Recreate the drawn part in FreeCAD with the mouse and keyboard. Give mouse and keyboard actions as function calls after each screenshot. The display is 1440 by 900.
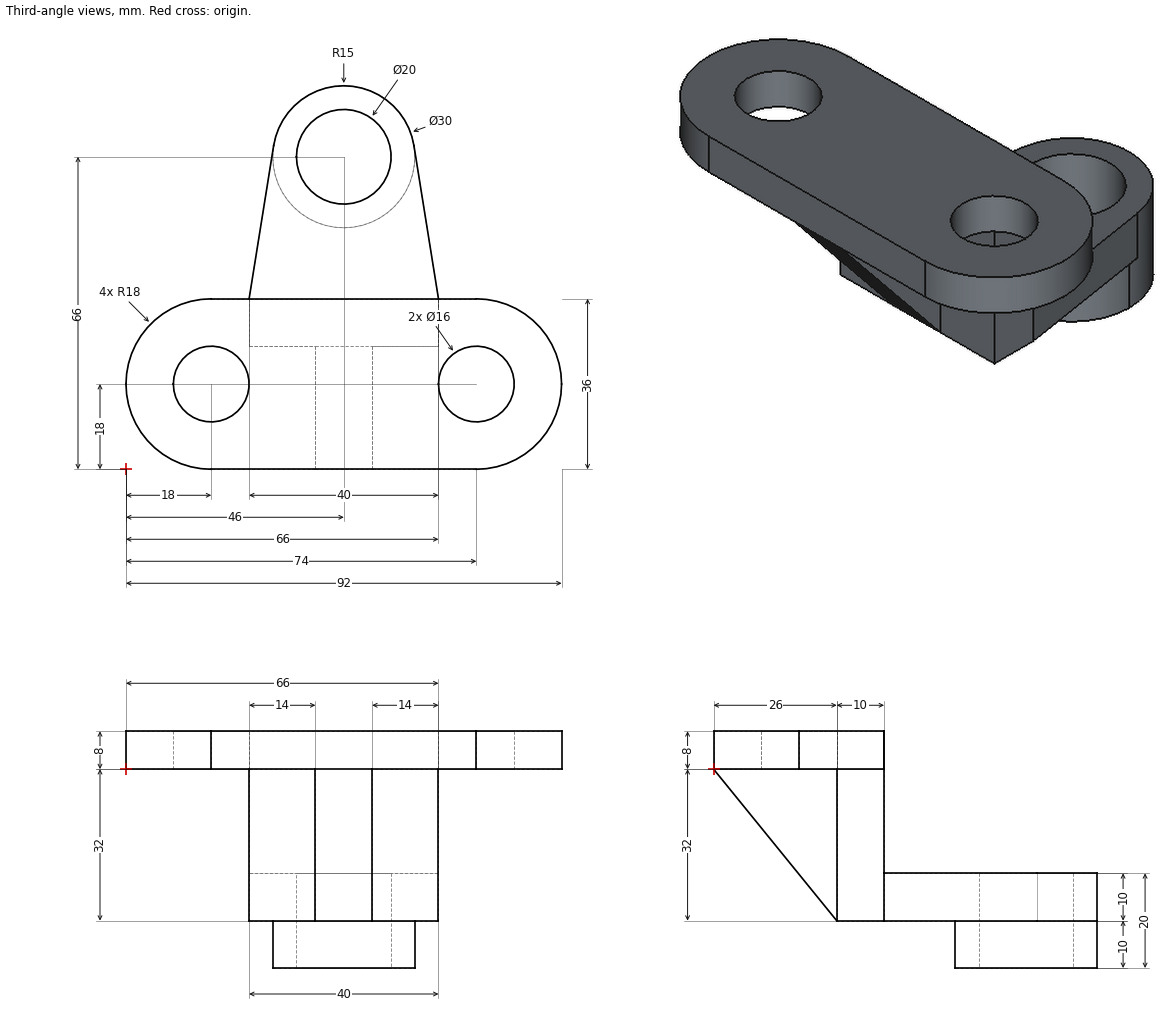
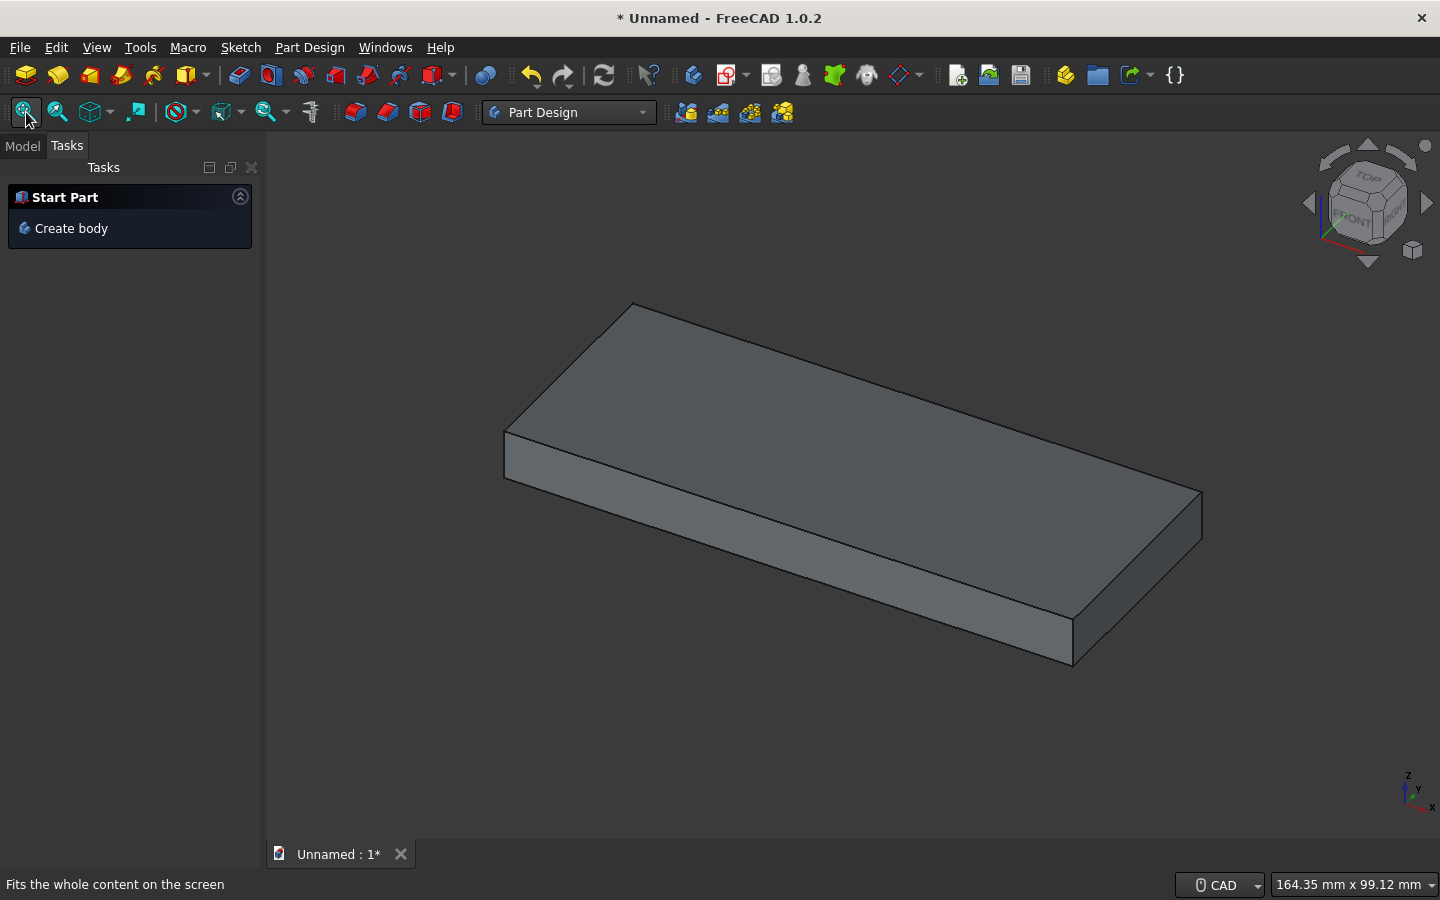
click(1016, 514)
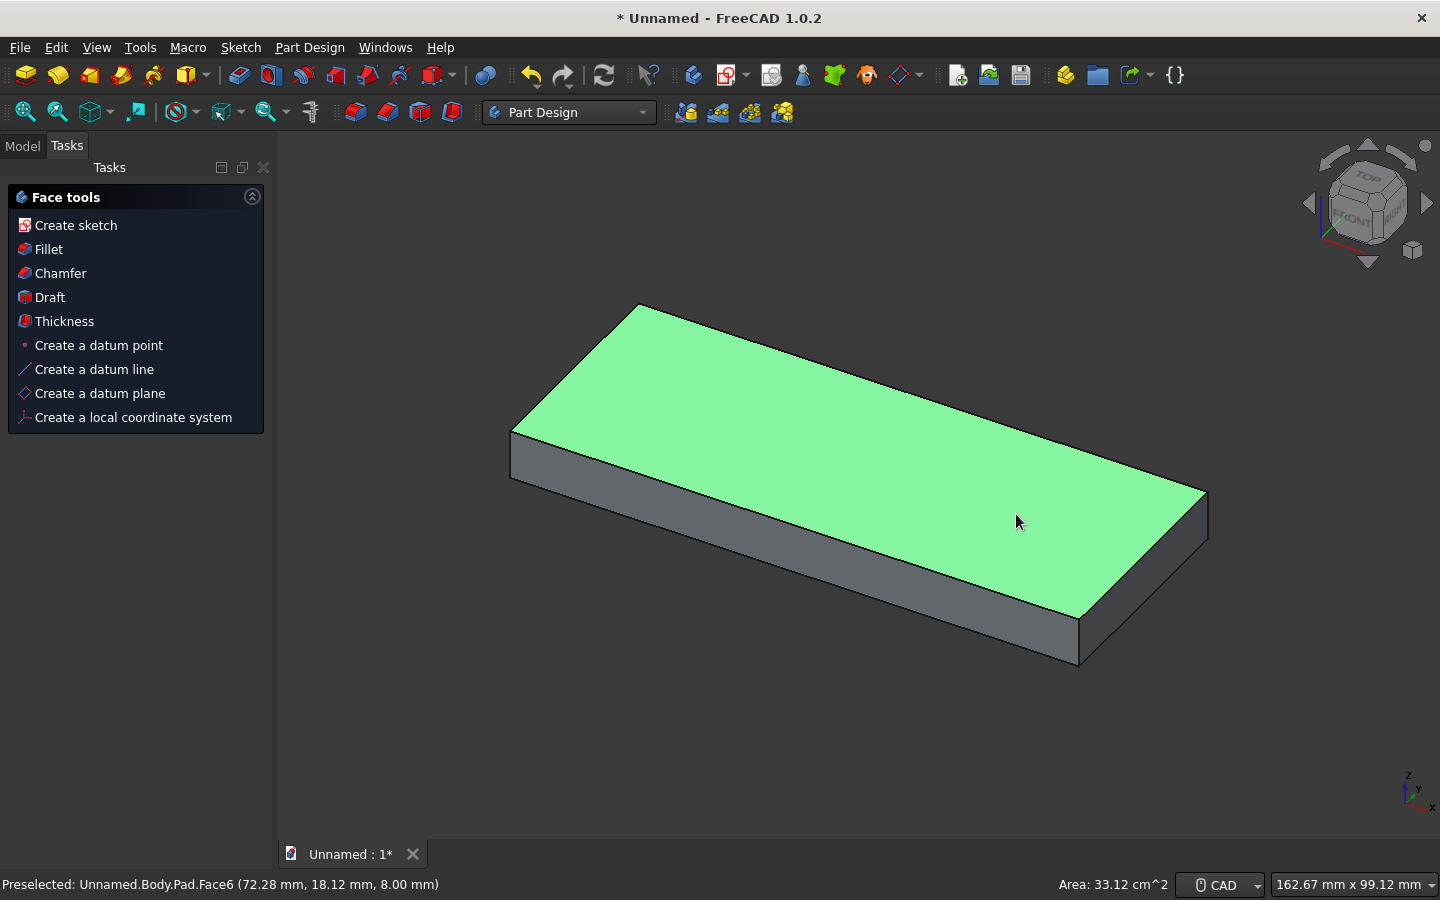
click(726, 76)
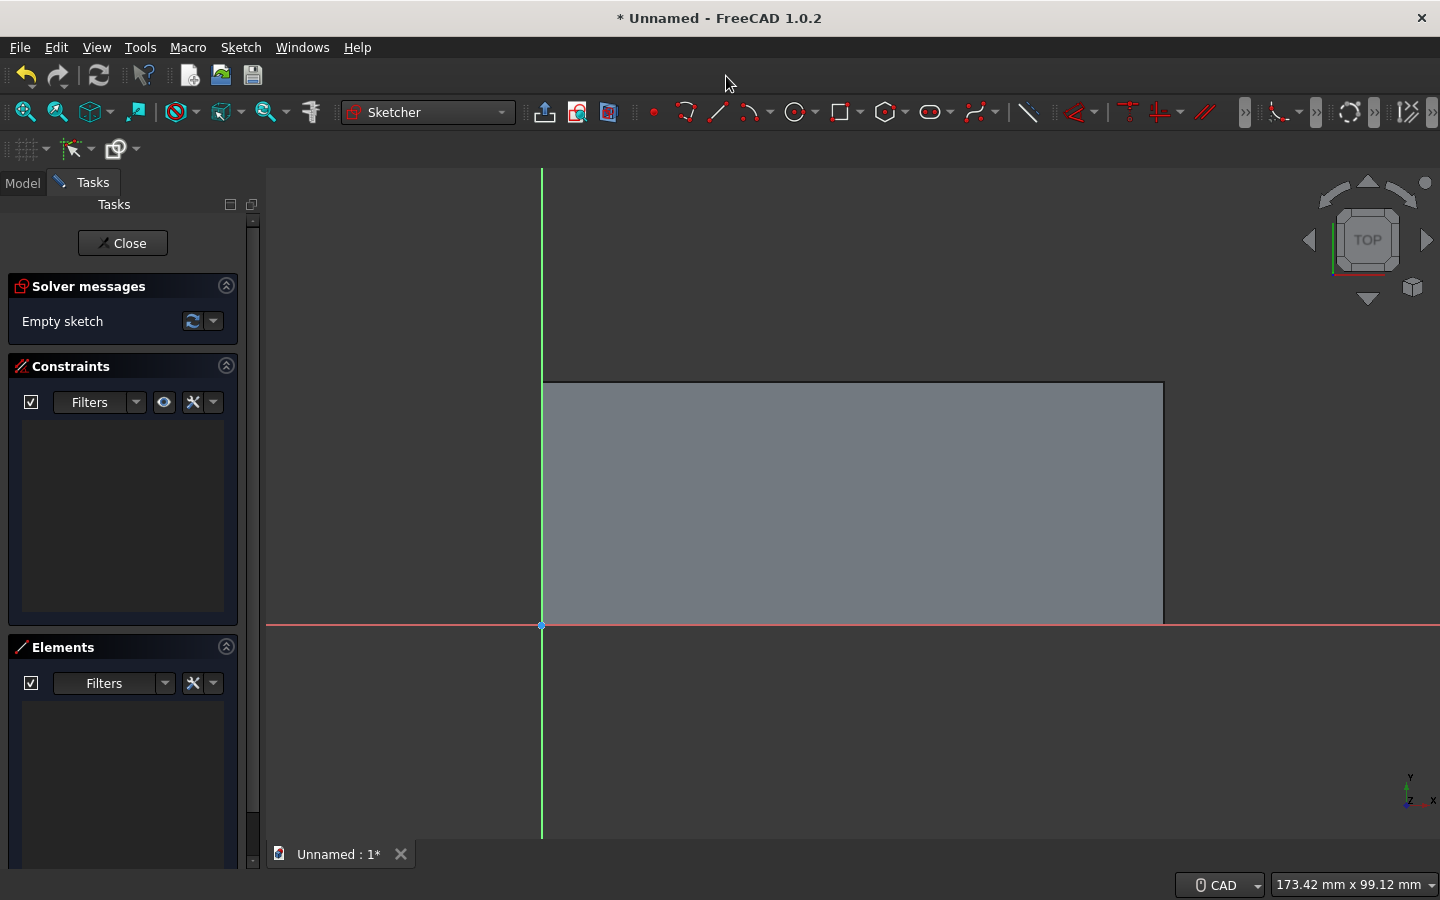
click(686, 112)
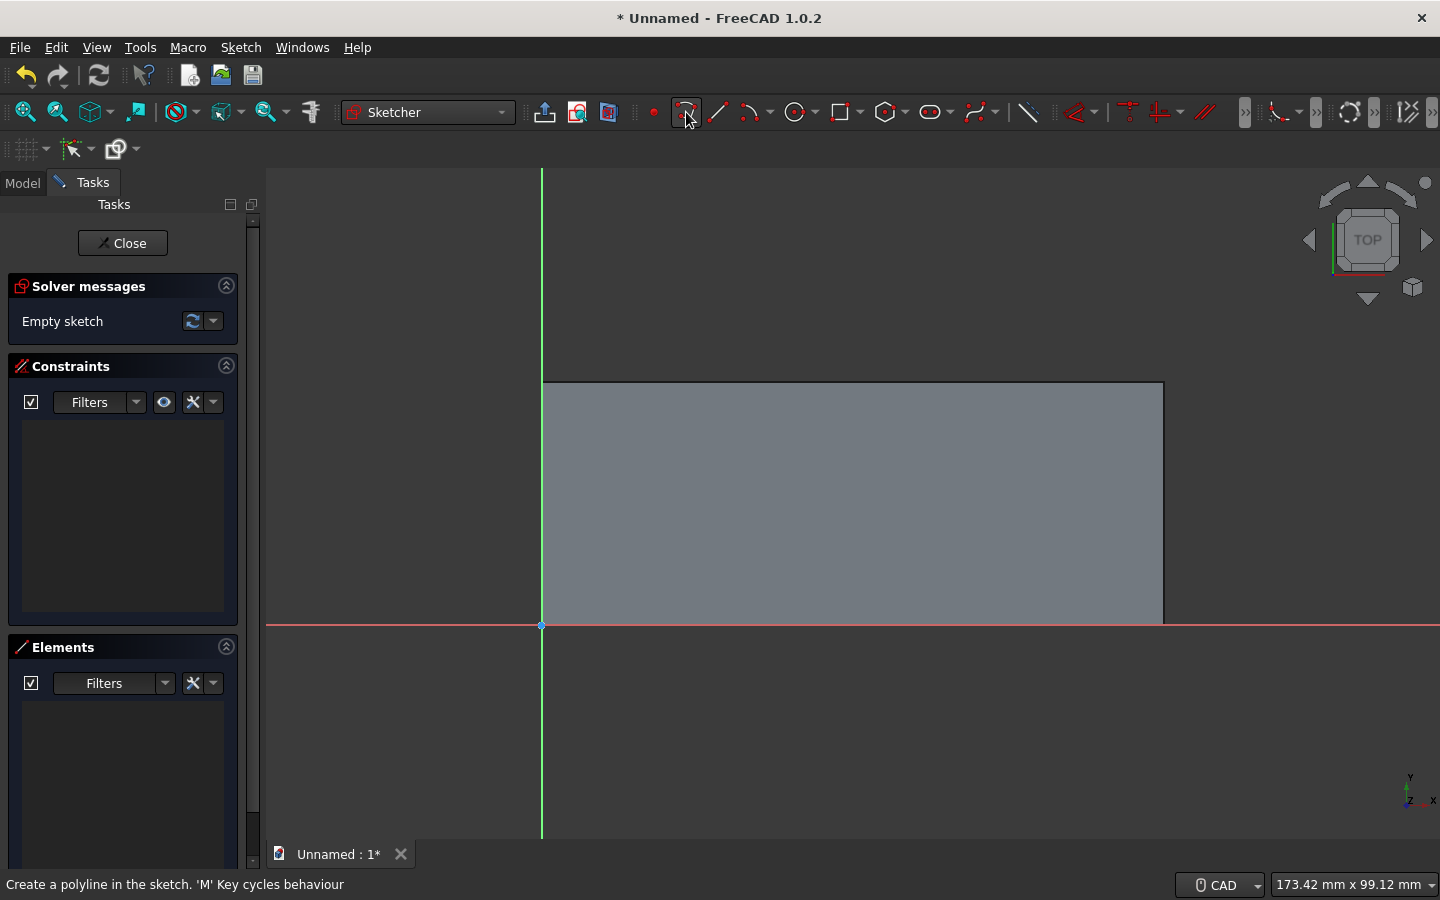
click(663, 382)
click(542, 382)
click(551, 504)
right_click(551, 504)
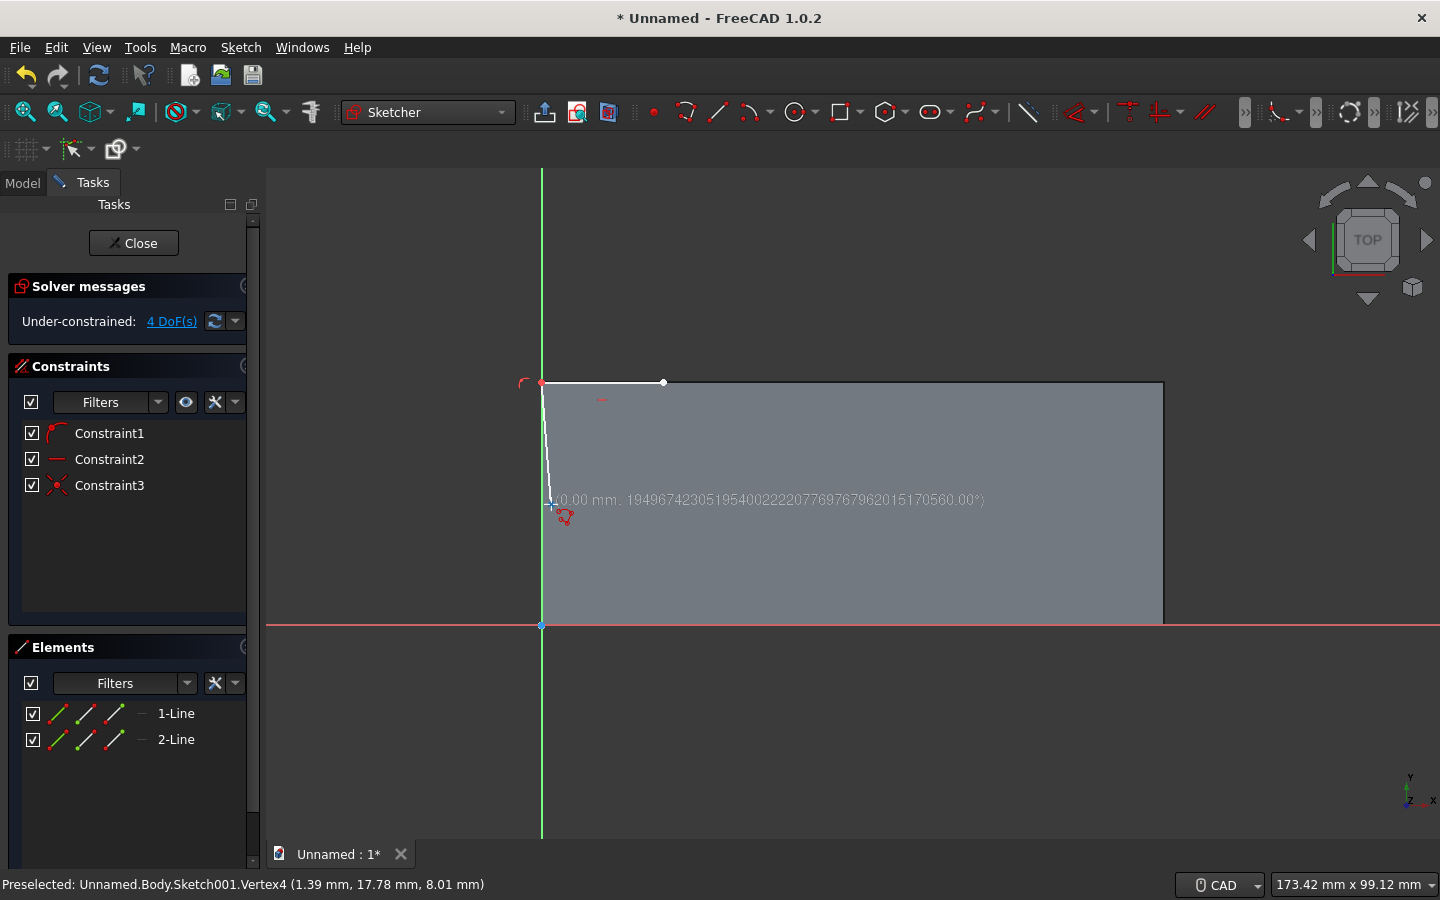
key(g)
key(3)
key(a)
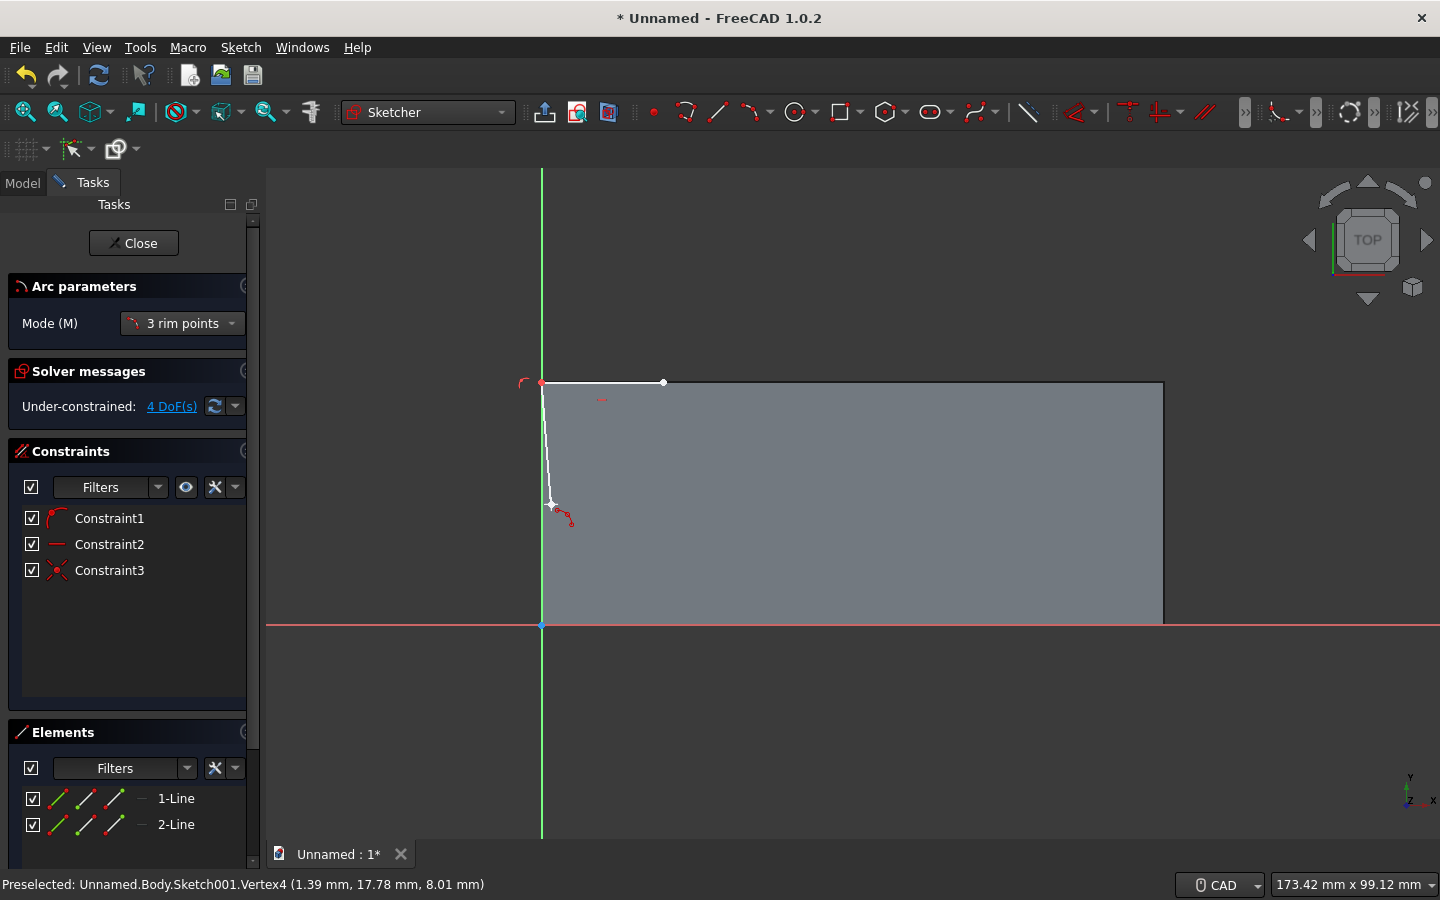
click(551, 505)
click(663, 383)
click(577, 417)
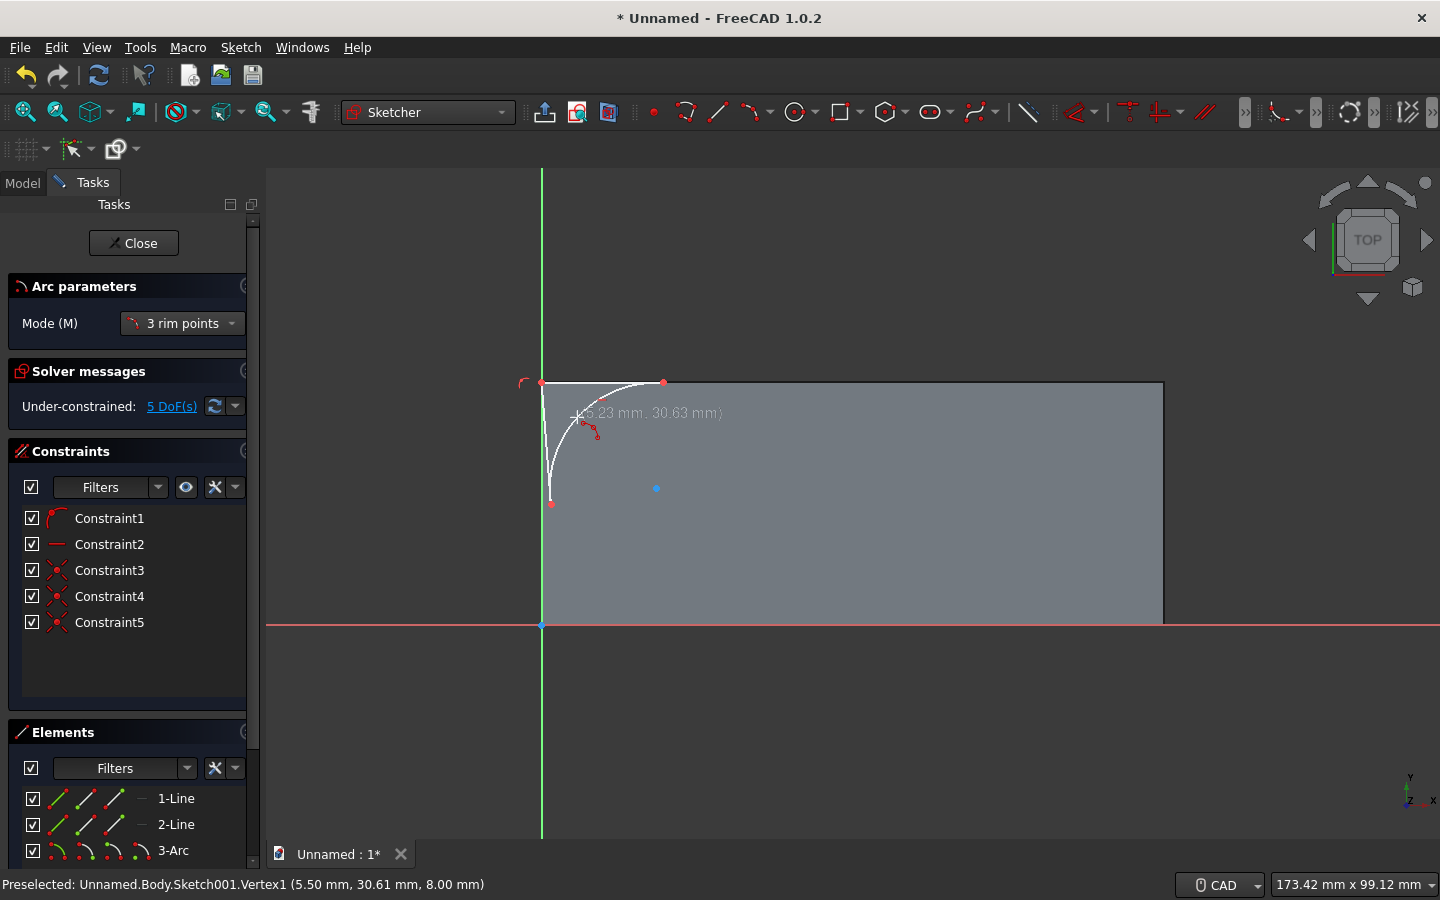
click(686, 112)